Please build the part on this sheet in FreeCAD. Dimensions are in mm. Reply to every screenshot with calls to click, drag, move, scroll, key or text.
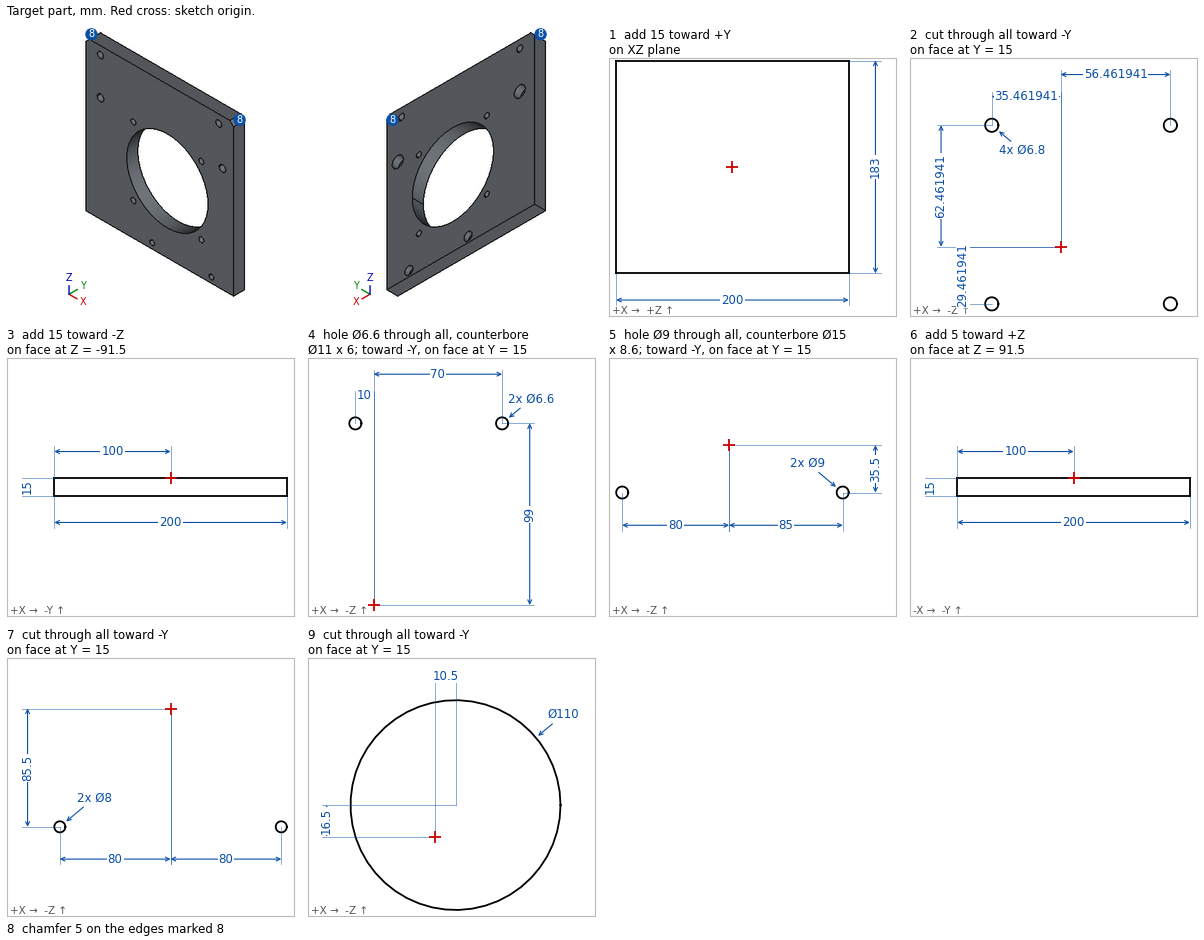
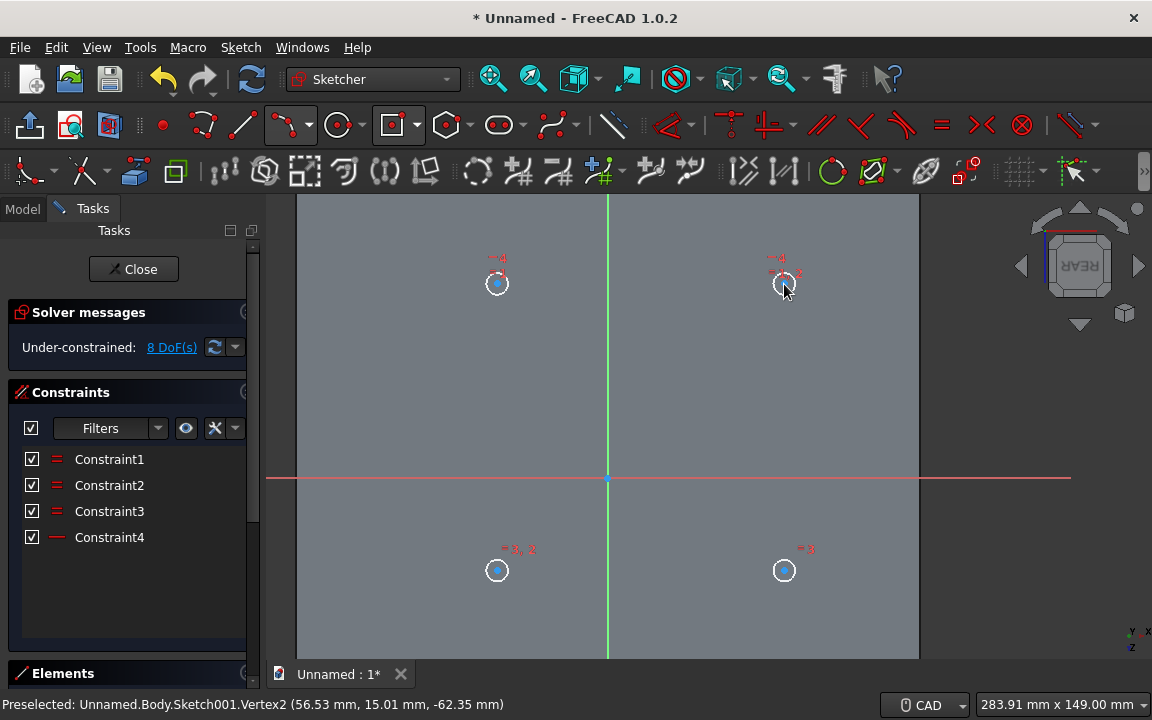
click(497, 284)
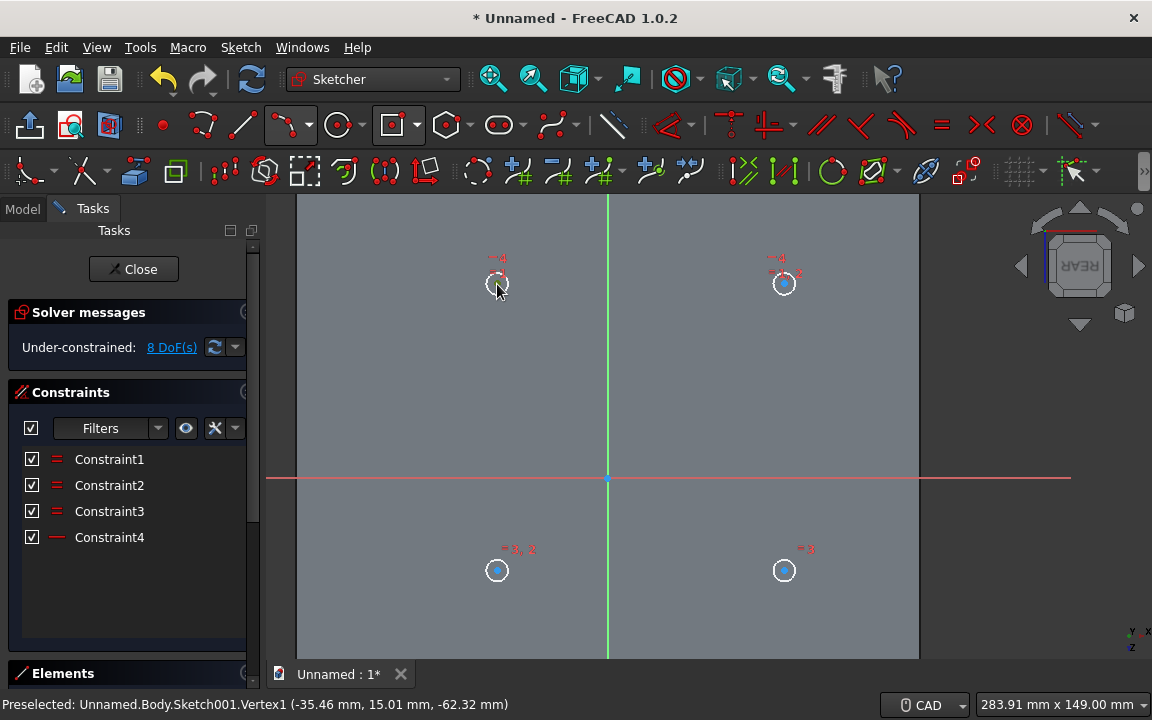
click(497, 571)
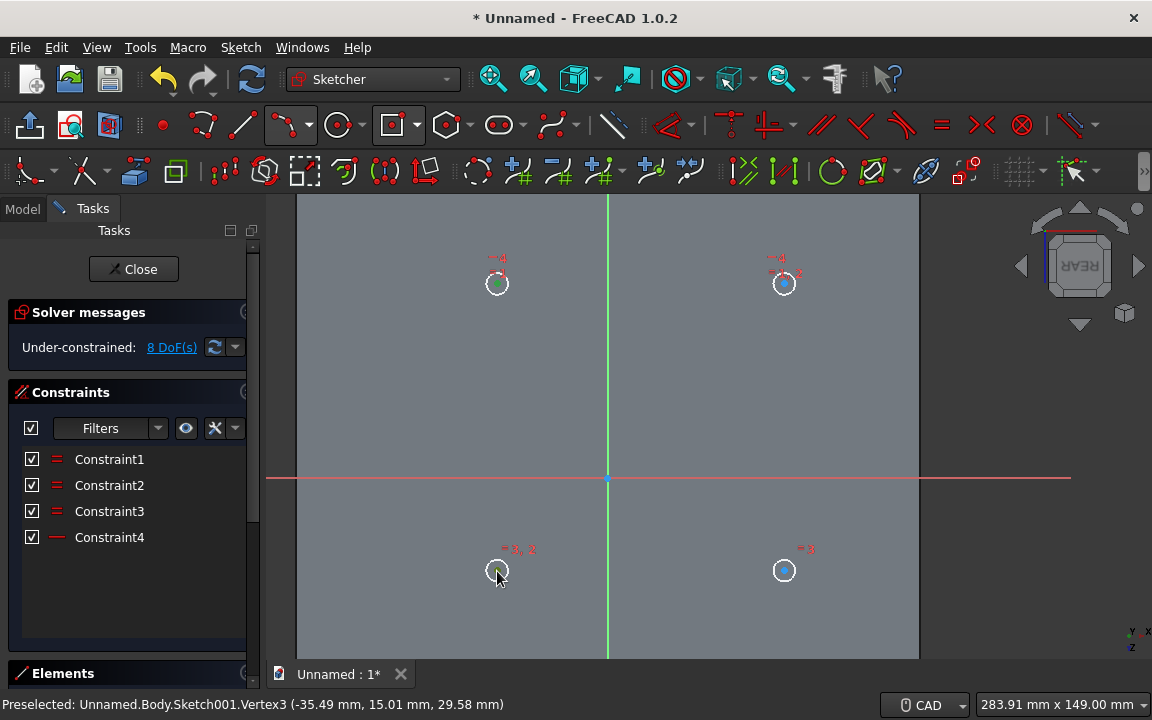
key(v)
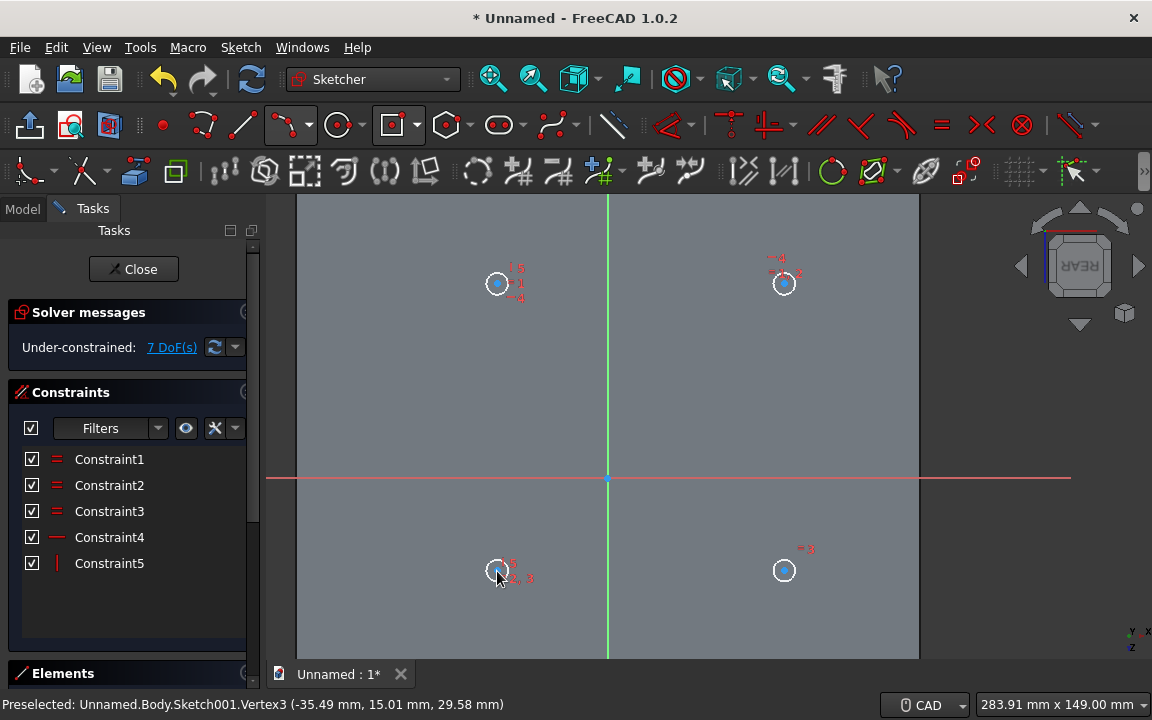
click(784, 284)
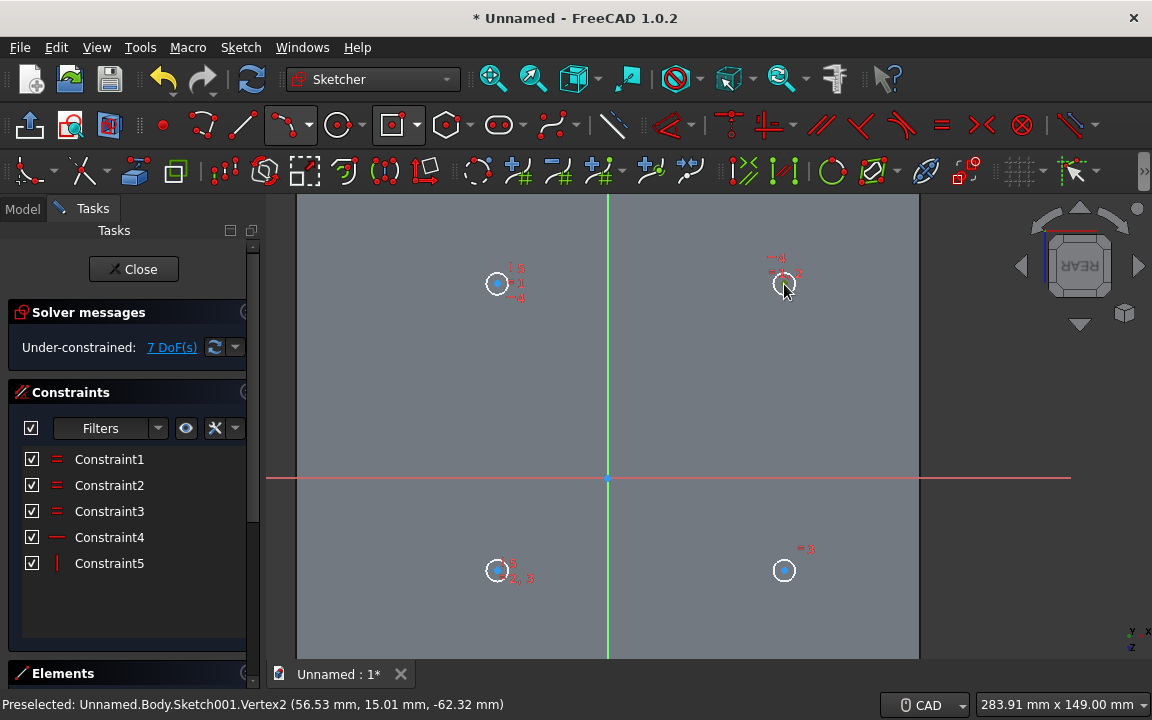
click(784, 571)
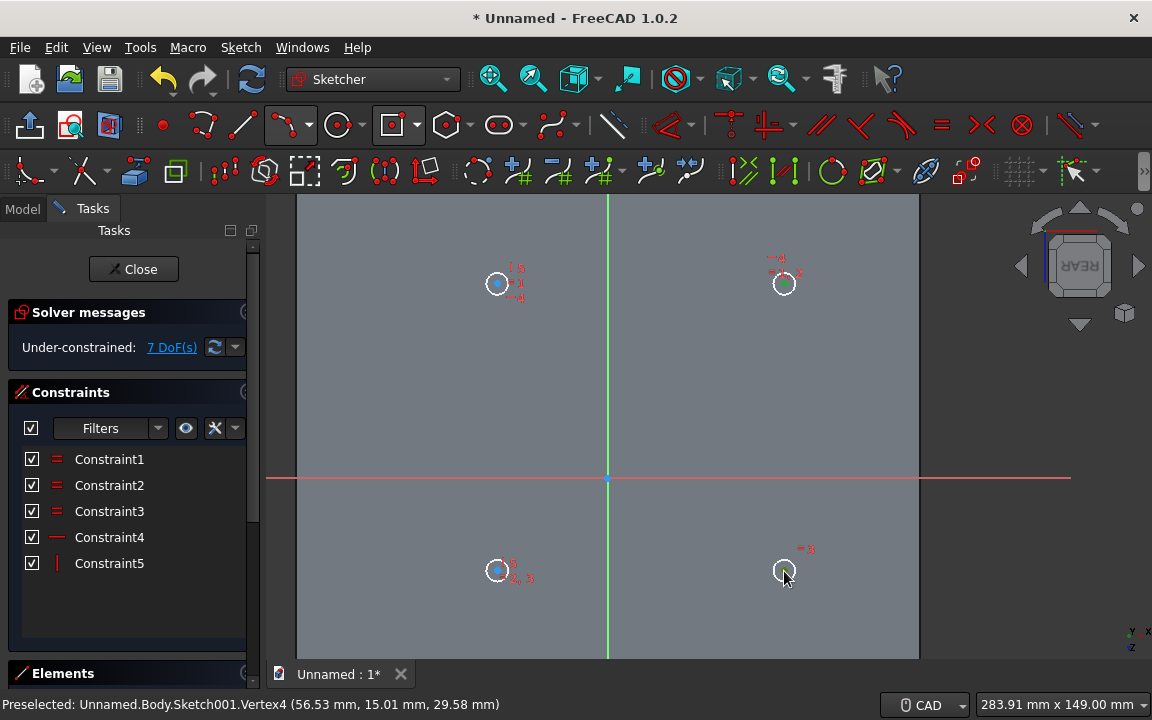
click(796, 126)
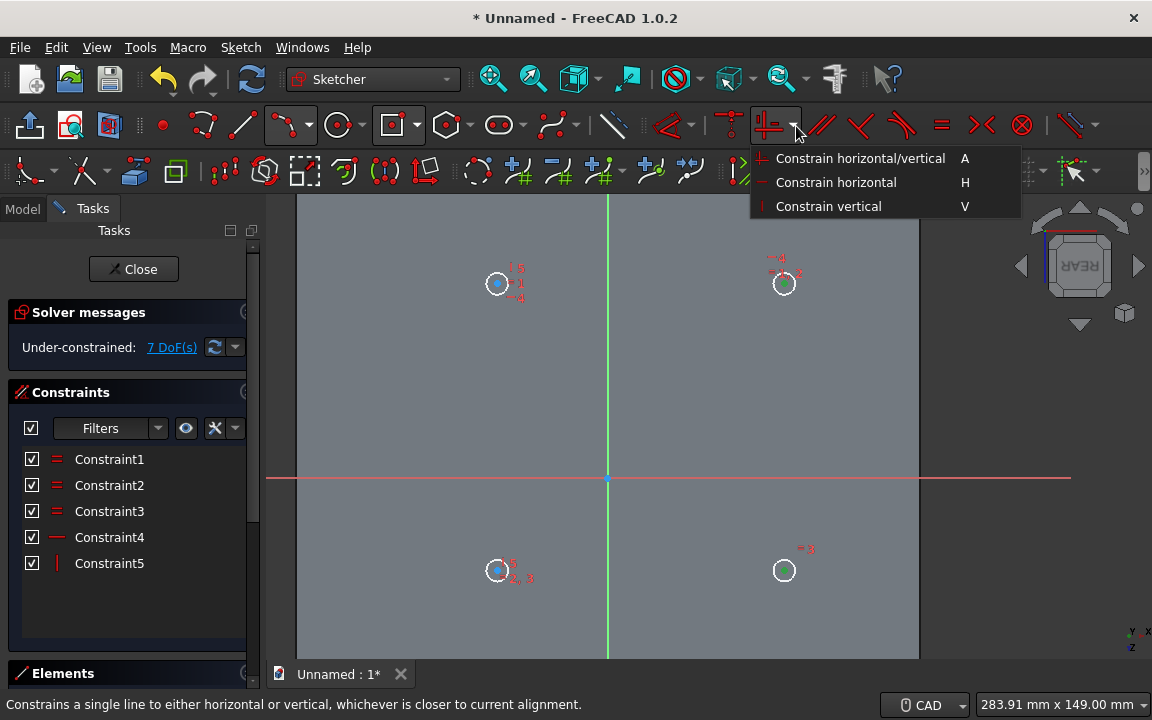
click(886, 206)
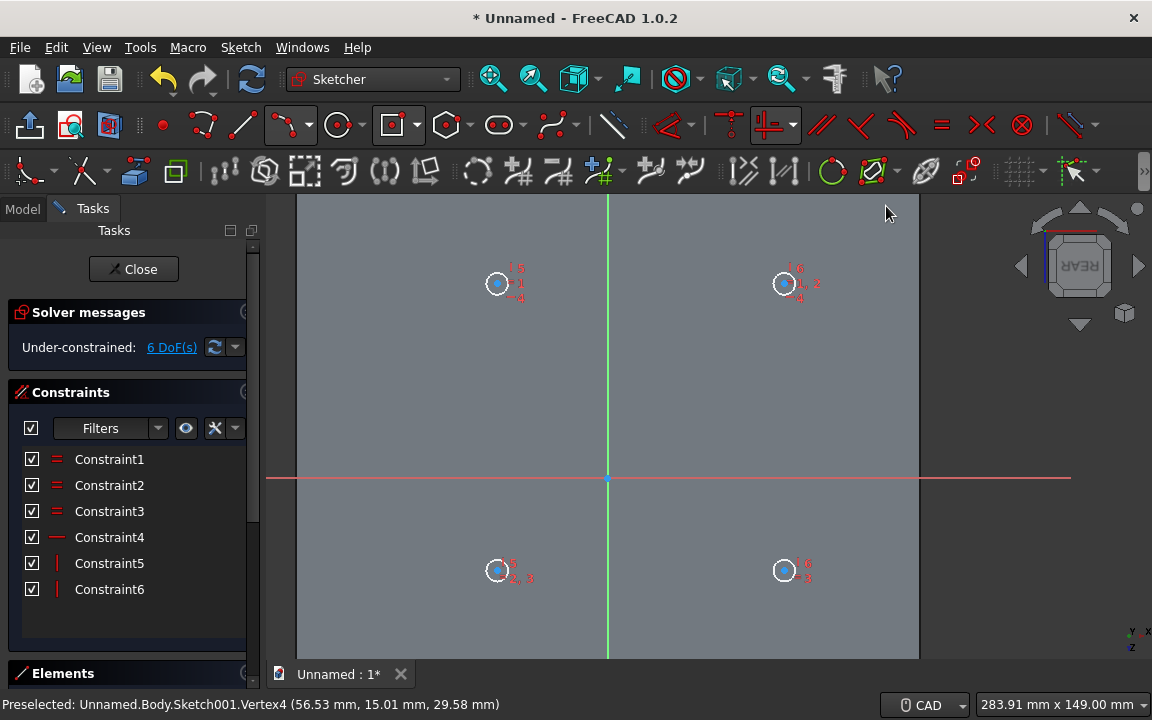
click(497, 571)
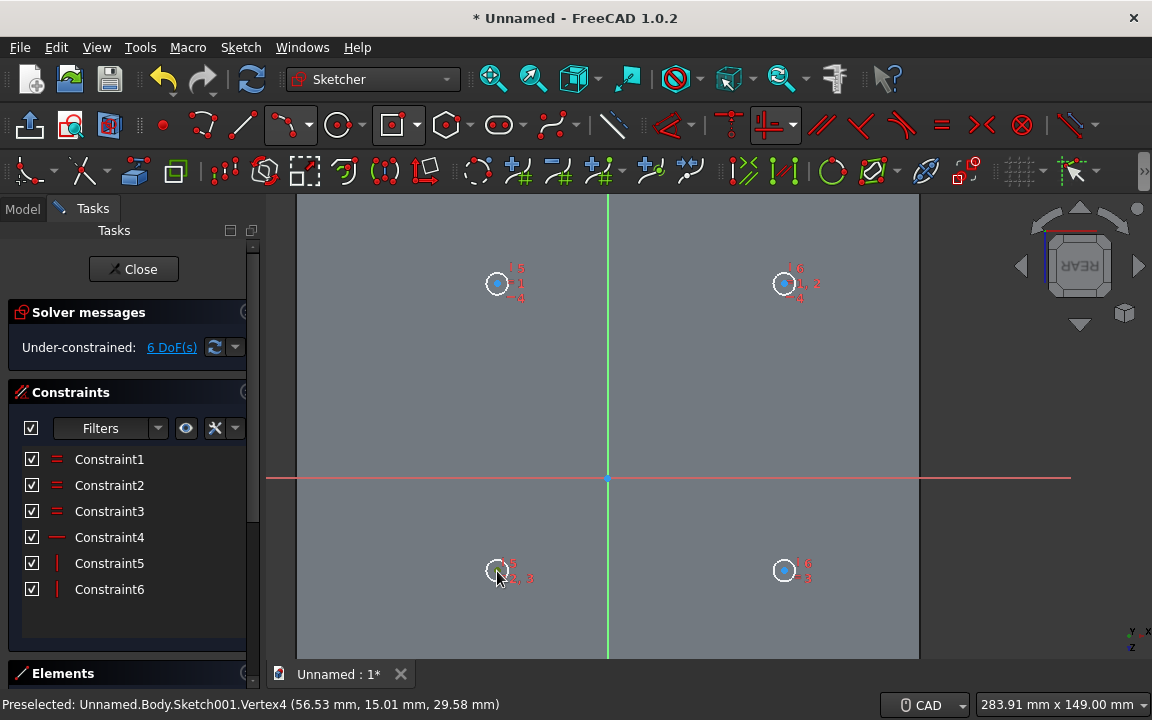
click(784, 571)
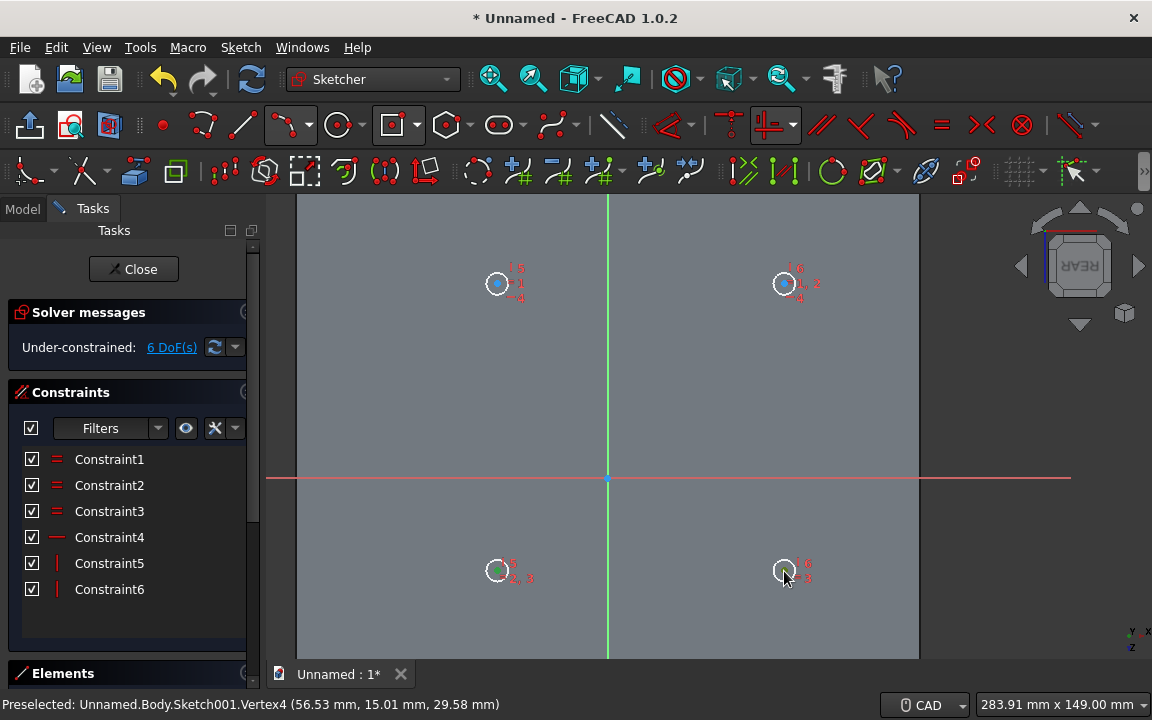
click(796, 126)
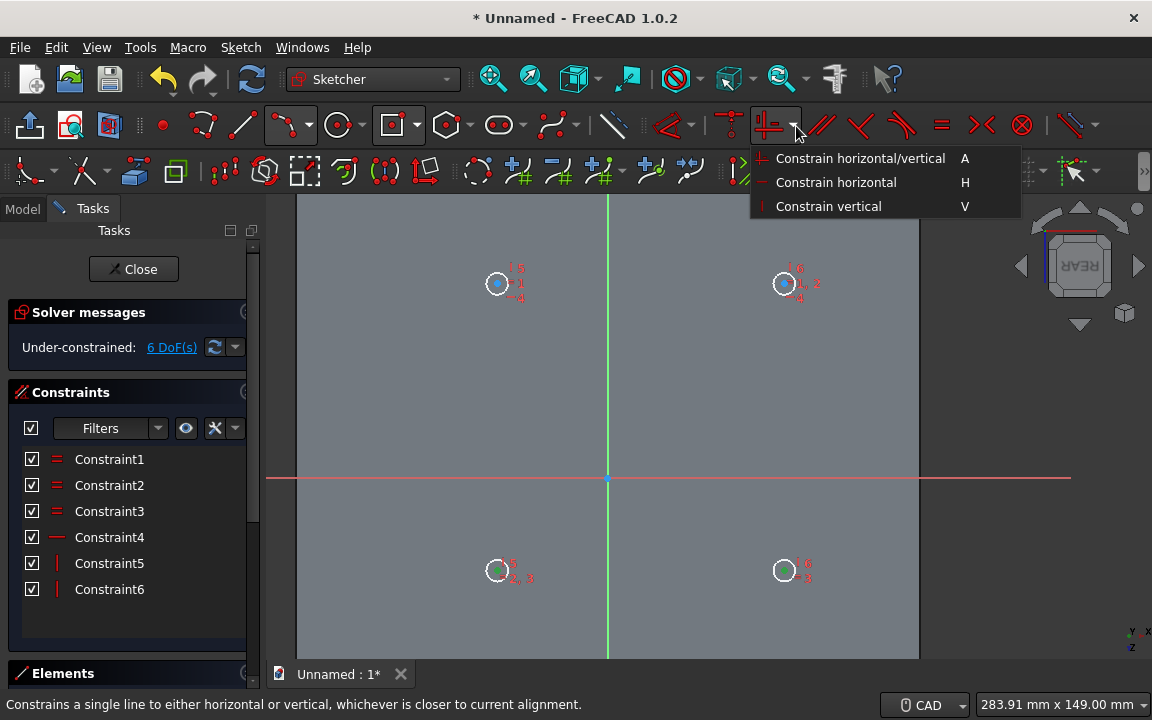
click(886, 182)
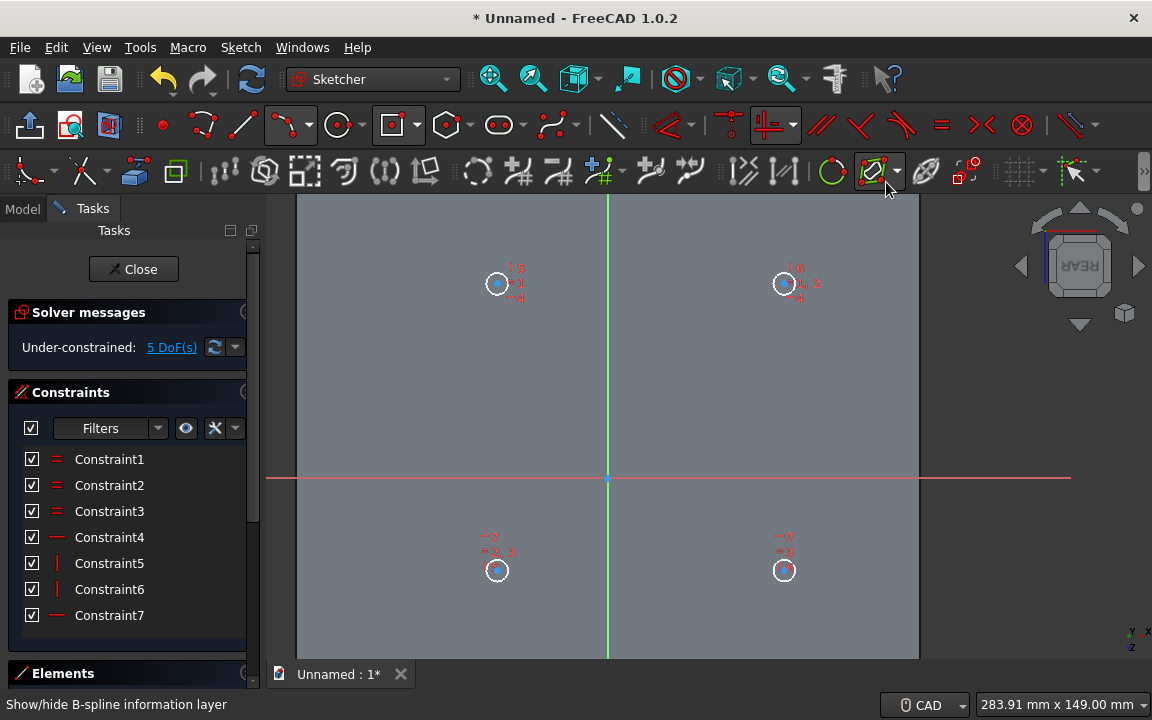
click(668, 126)